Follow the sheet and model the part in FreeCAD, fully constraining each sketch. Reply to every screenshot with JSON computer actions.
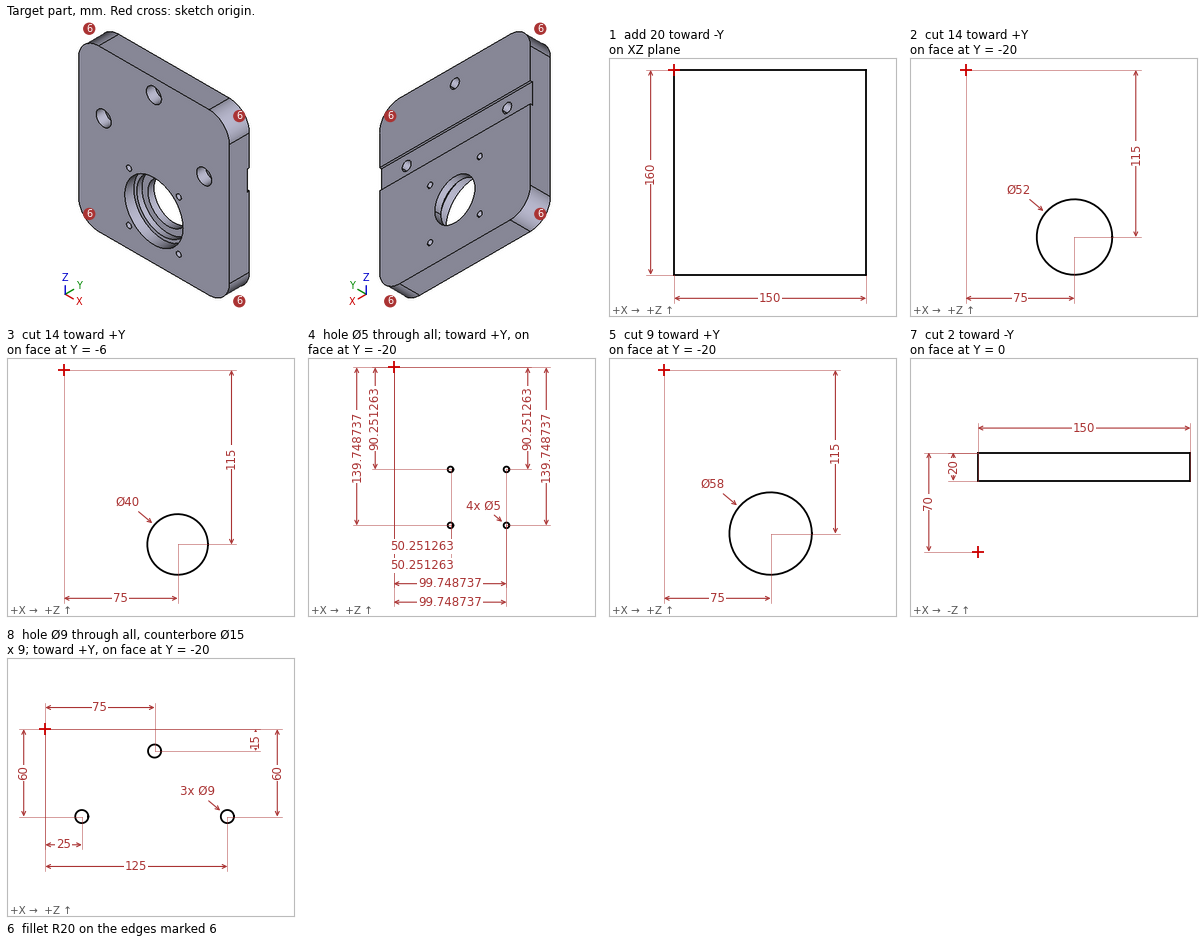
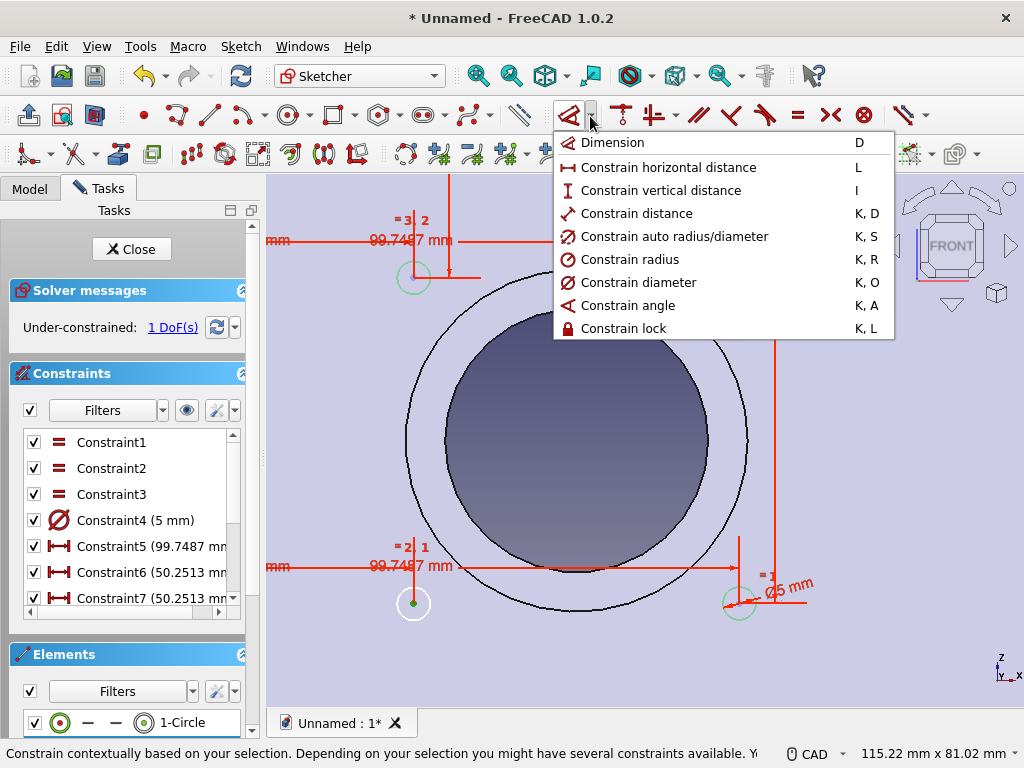
{"action": "left_click", "coordinate": [724, 190]}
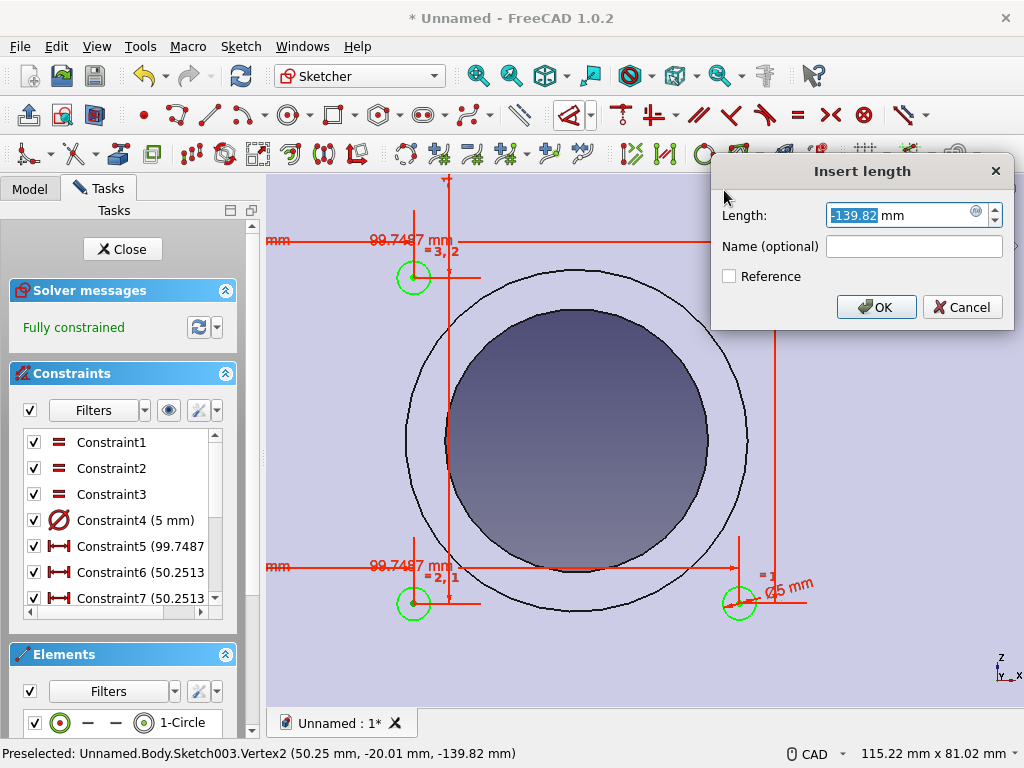
{"action": "type", "text": "-139.748737"}
{"action": "key", "text": "Return"}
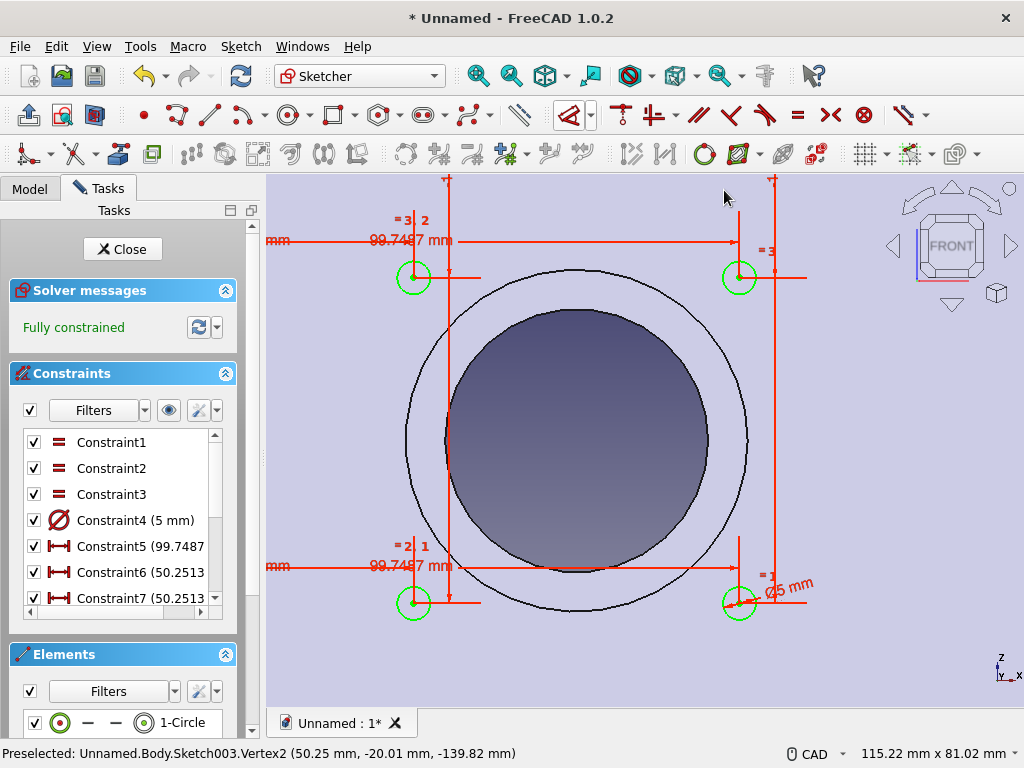
{"action": "left_click", "coordinate": [123, 249]}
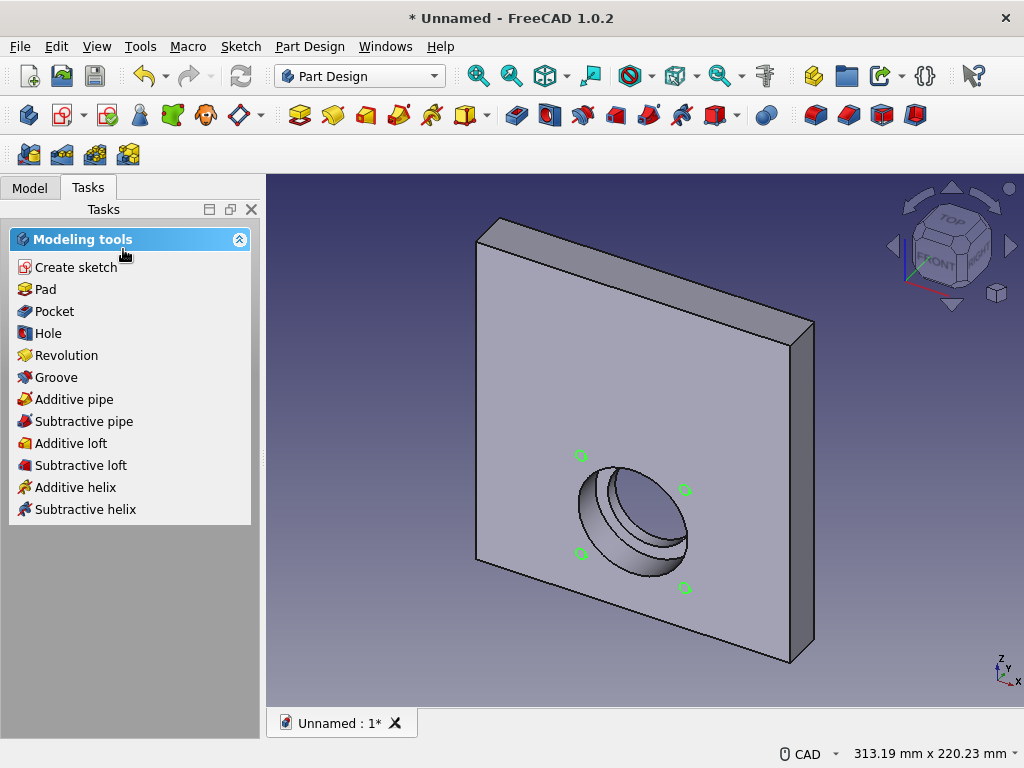
{"action": "left_click", "coordinate": [550, 116]}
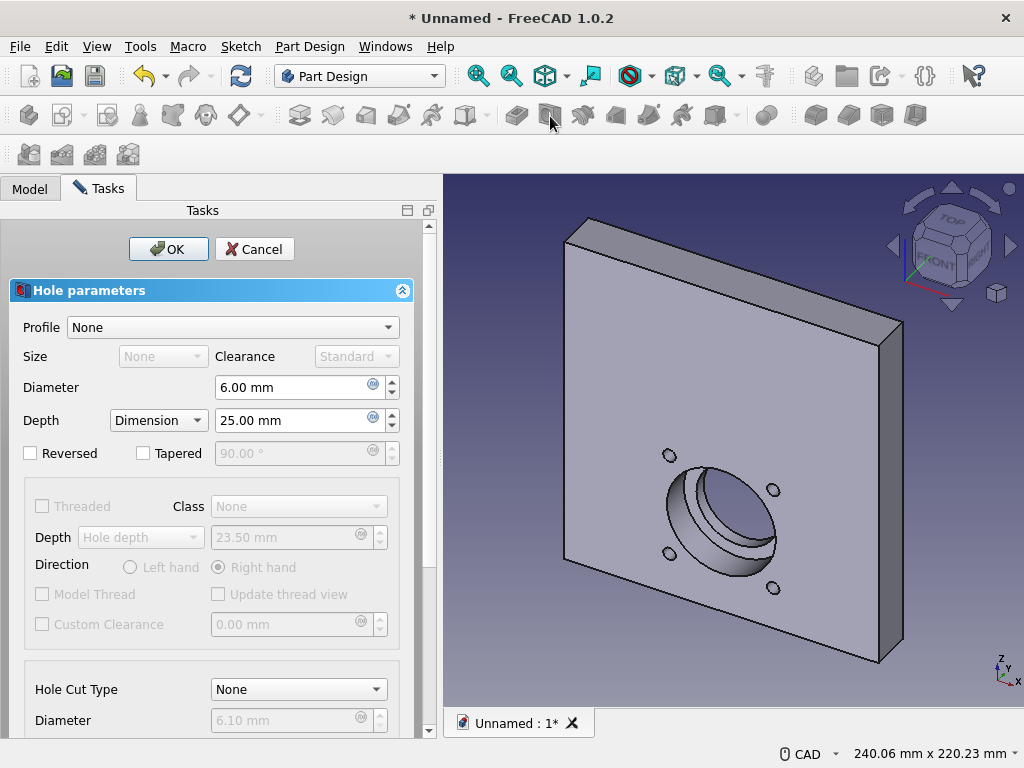
{"action": "triple_click", "coordinate": [300, 388]}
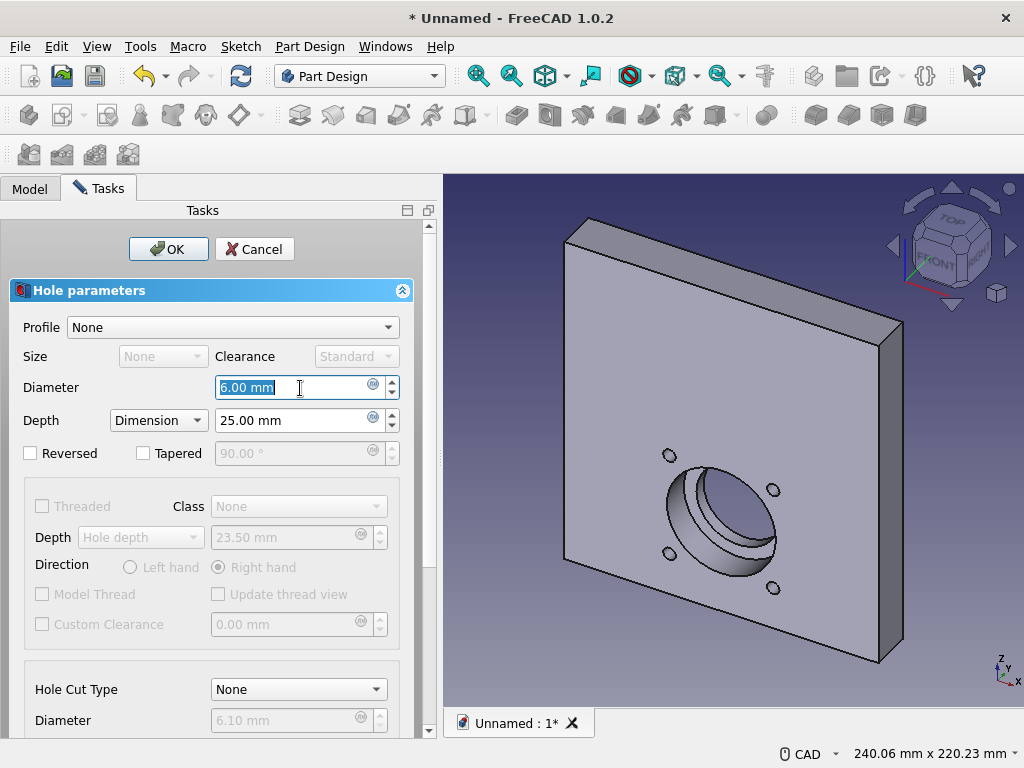
{"action": "type", "text": "5"}
{"action": "key", "text": "Tab"}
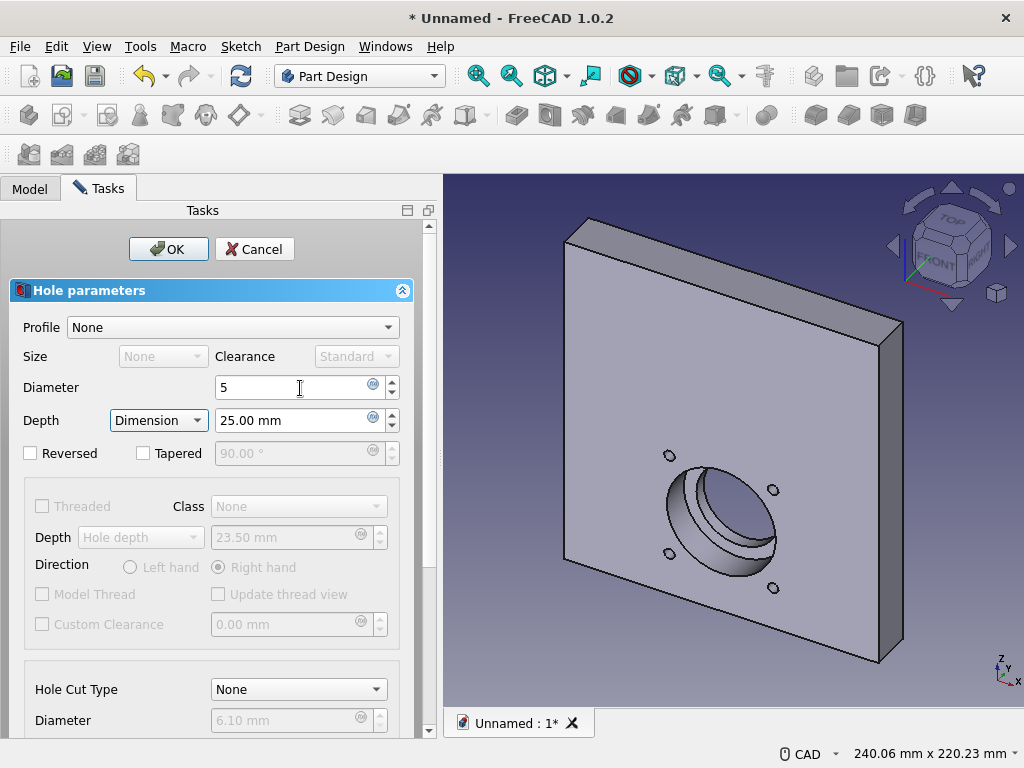
{"action": "left_click", "coordinate": [160, 420]}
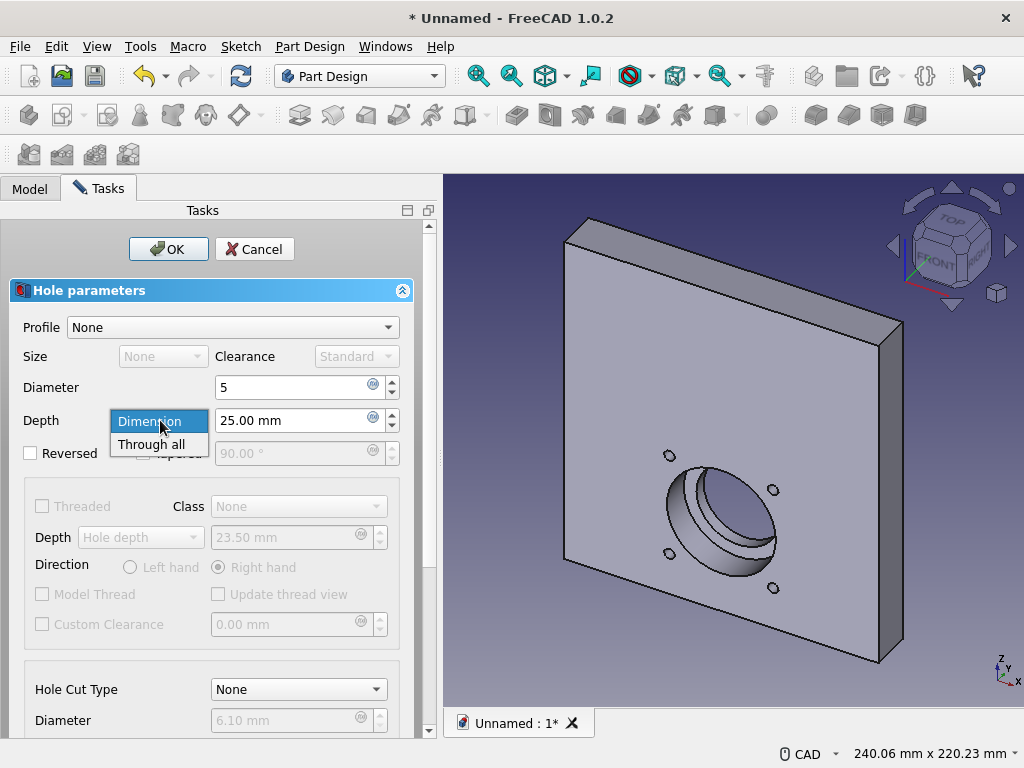
{"action": "left_click", "coordinate": [158, 444]}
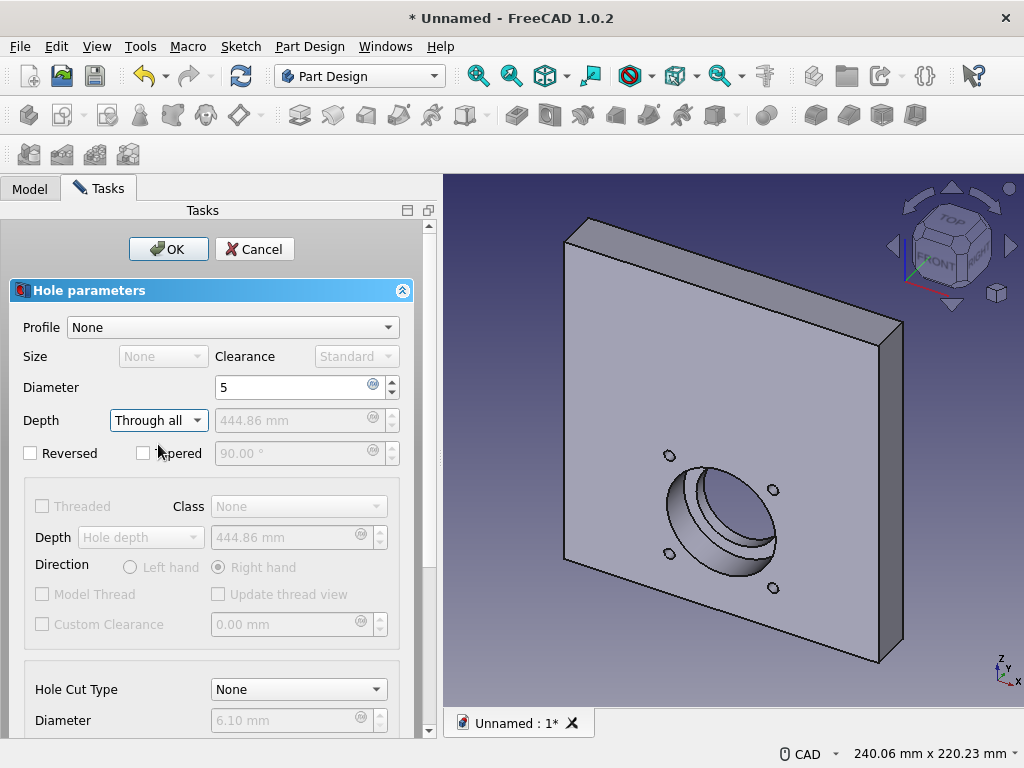
{"action": "left_click", "coordinate": [169, 249]}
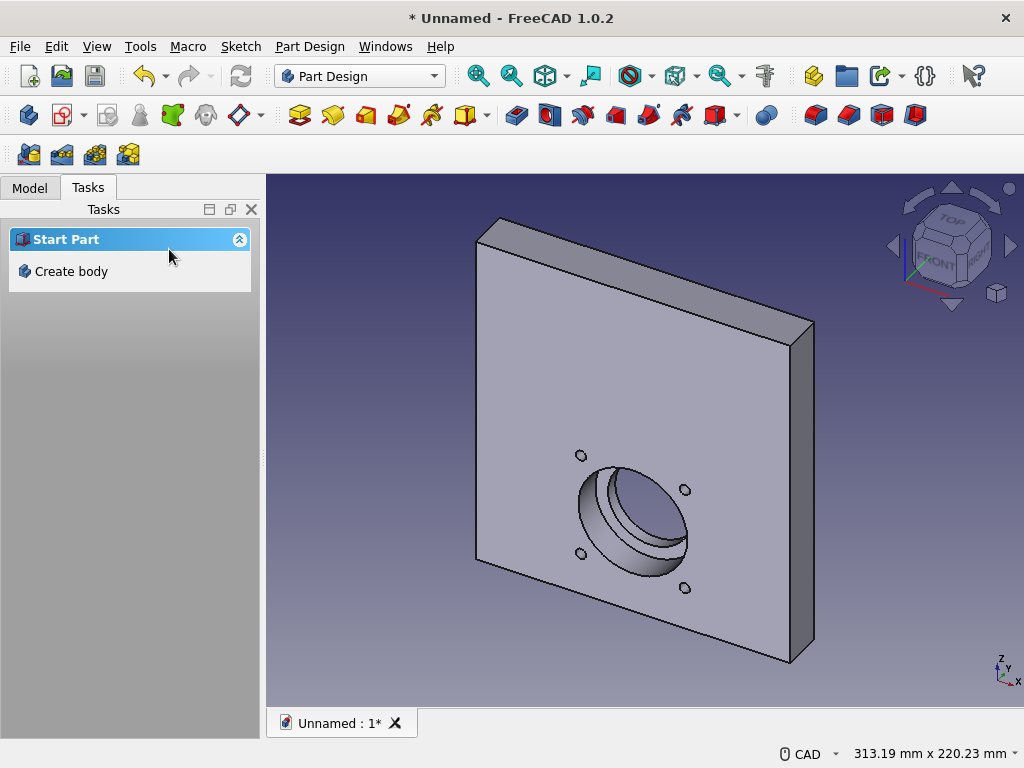
{"action": "left_click", "coordinate": [678, 376]}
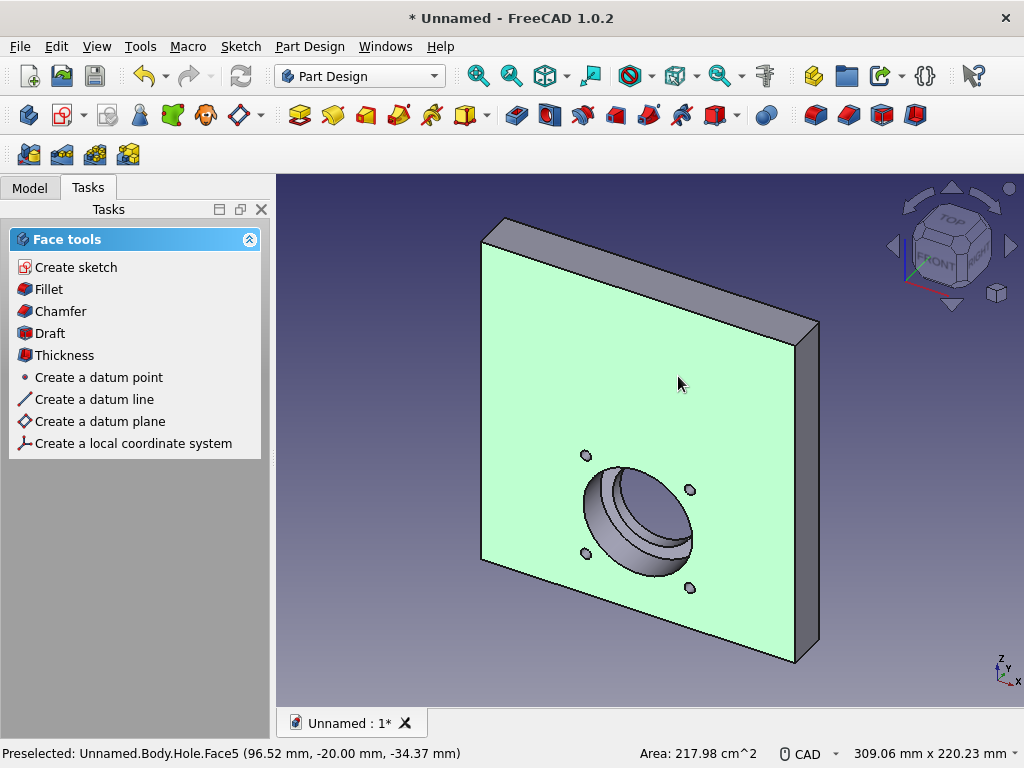
{"action": "left_click", "coordinate": [62, 116]}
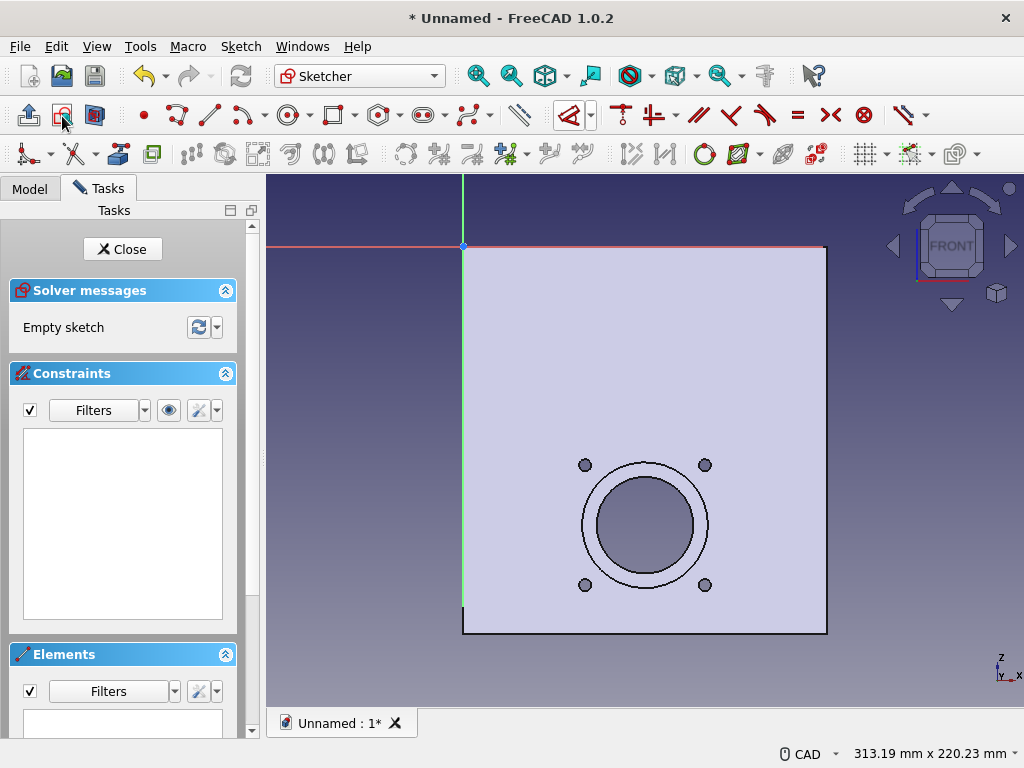
{"action": "left_click", "coordinate": [288, 116]}